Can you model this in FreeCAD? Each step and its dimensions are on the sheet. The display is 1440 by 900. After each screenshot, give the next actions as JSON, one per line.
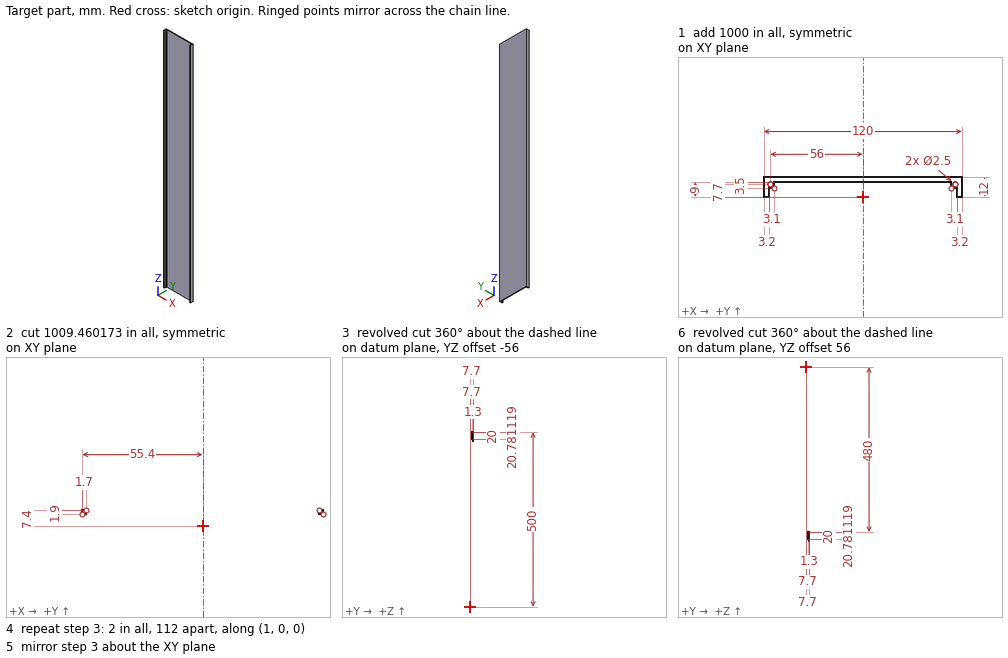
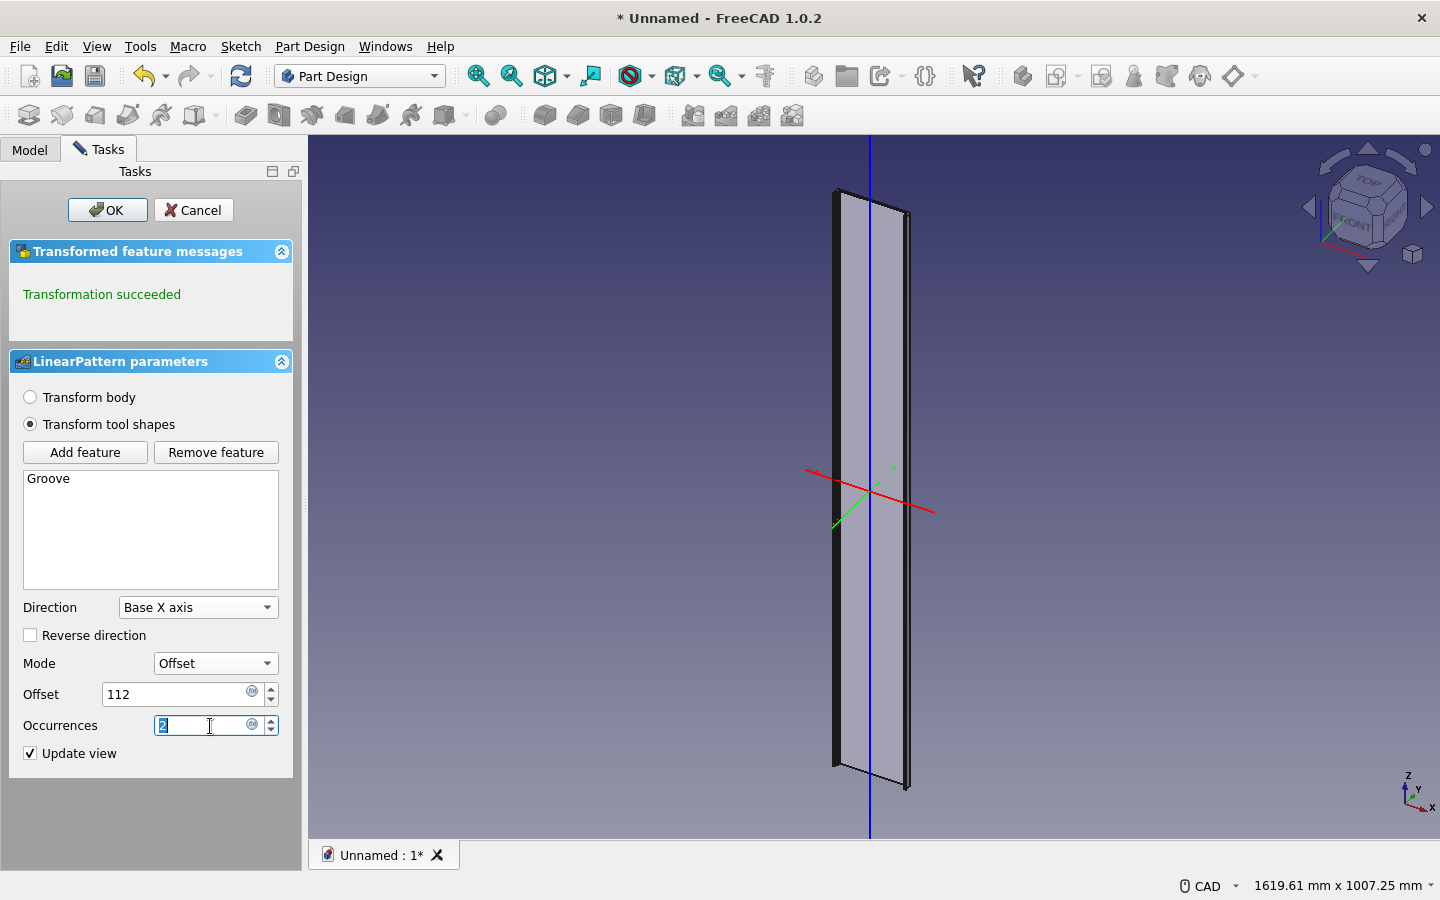
{"action": "type", "text": "2"}
{"action": "key", "text": "Tab"}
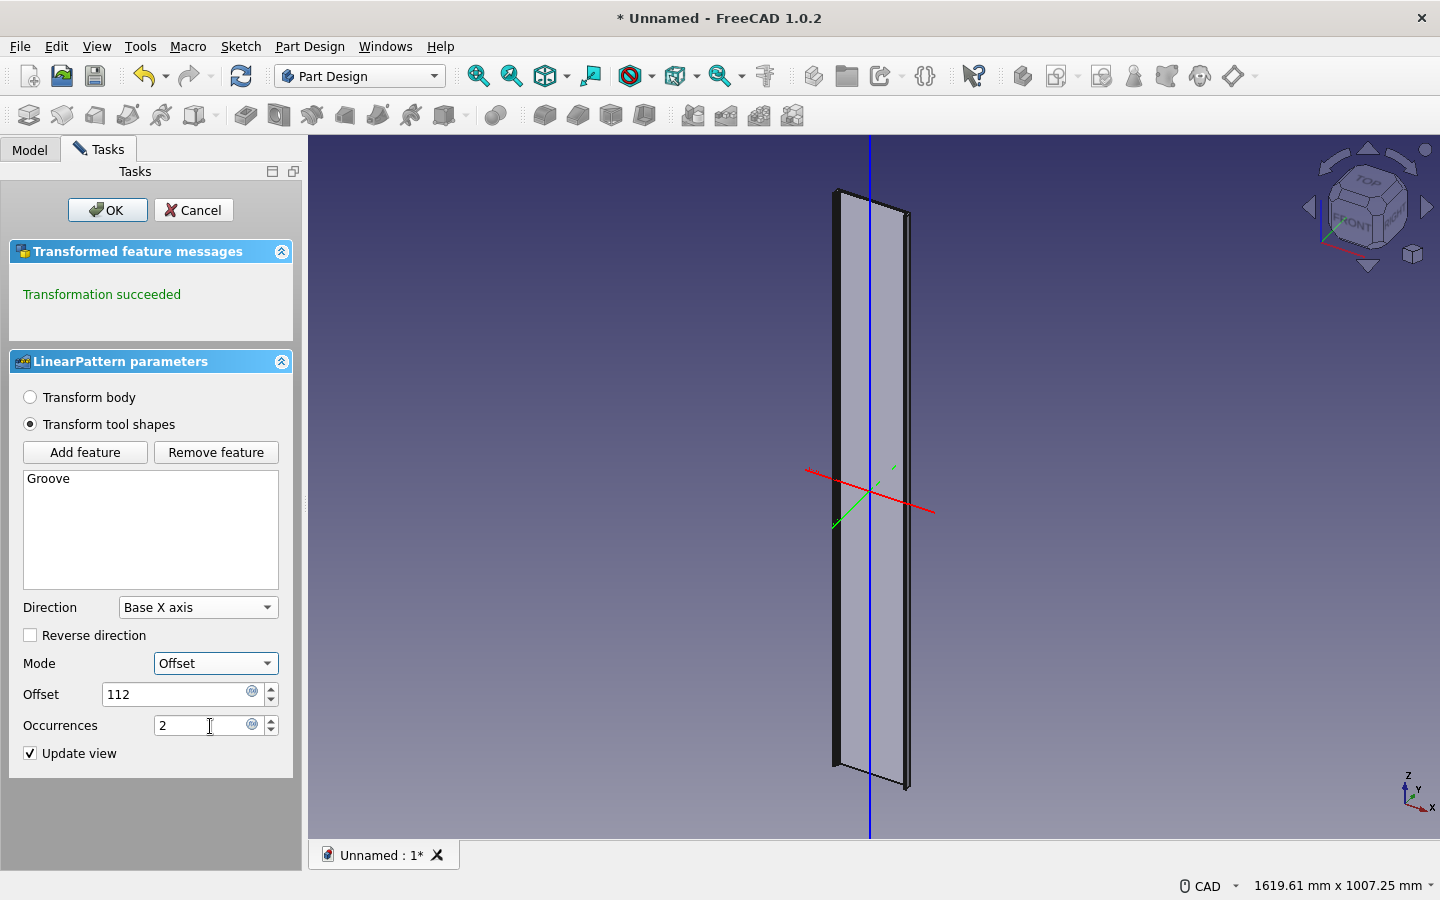
{"action": "left_click", "coordinate": [108, 210]}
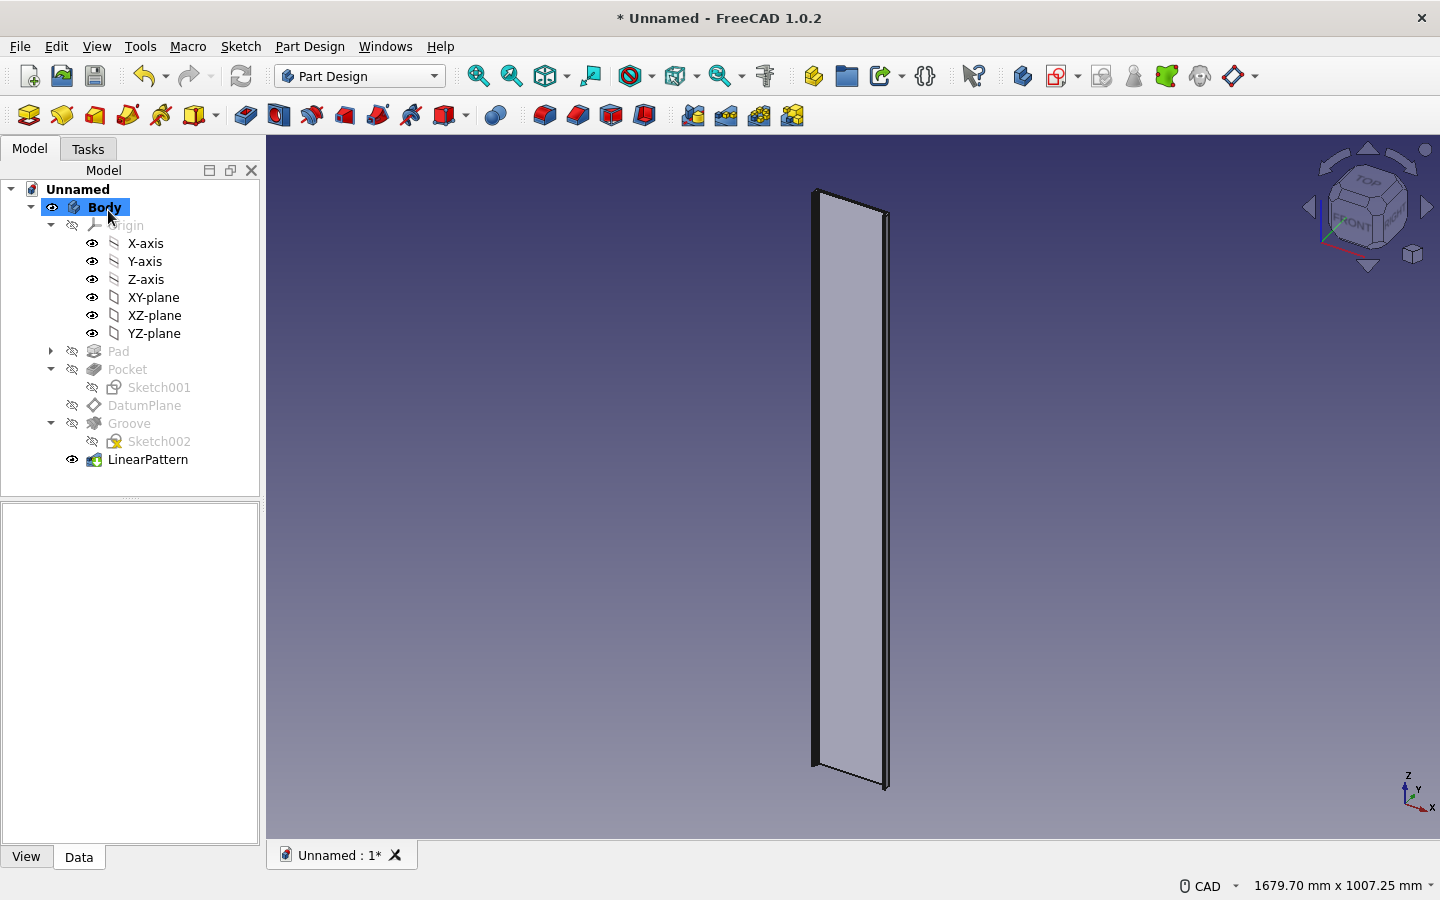
{"action": "left_click", "coordinate": [117, 423]}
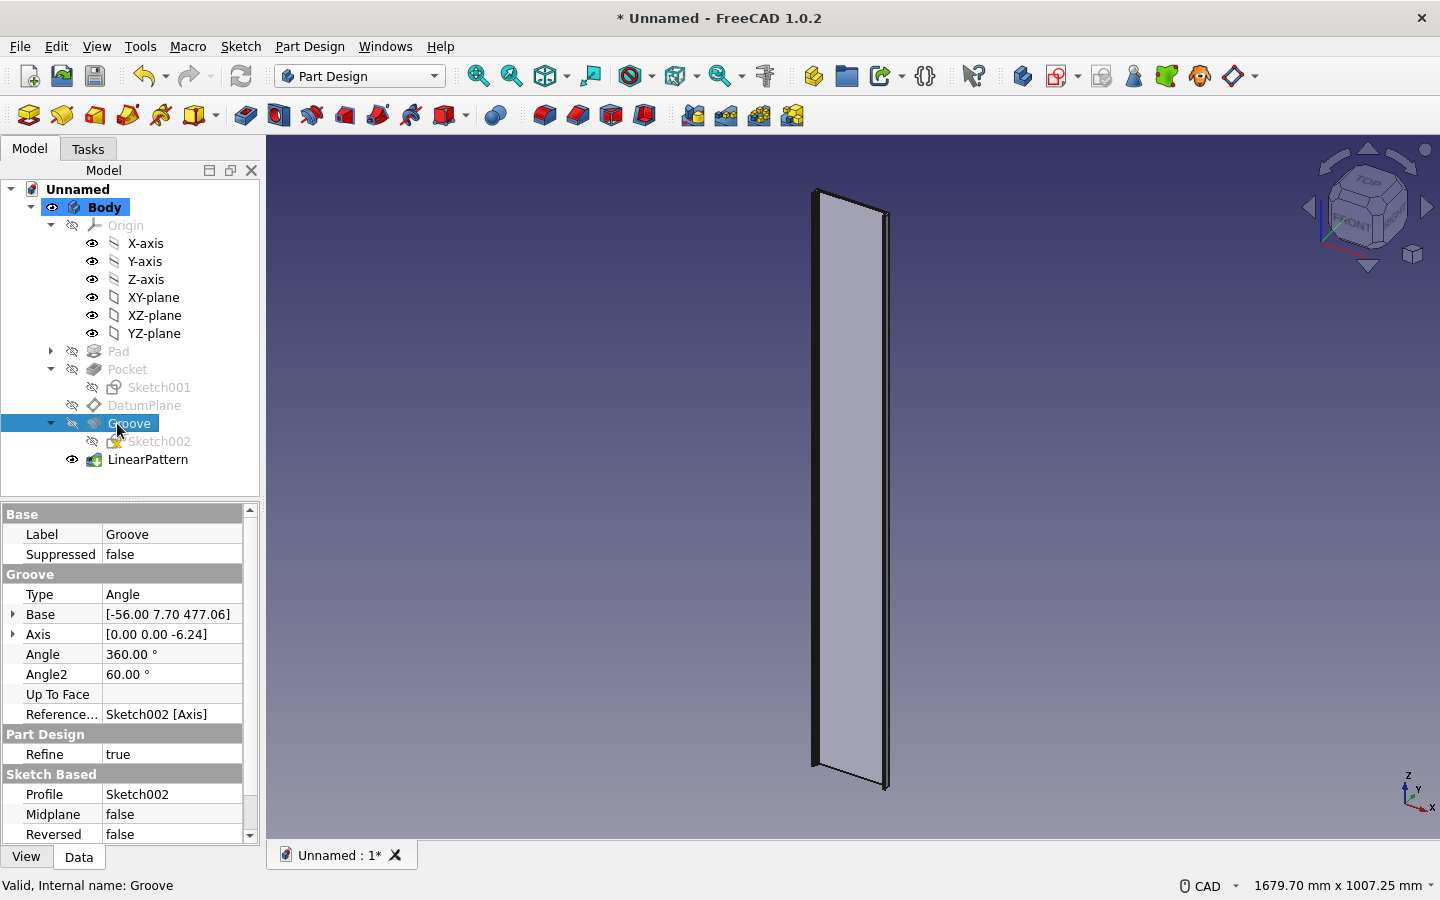
{"action": "left_click", "coordinate": [693, 116]}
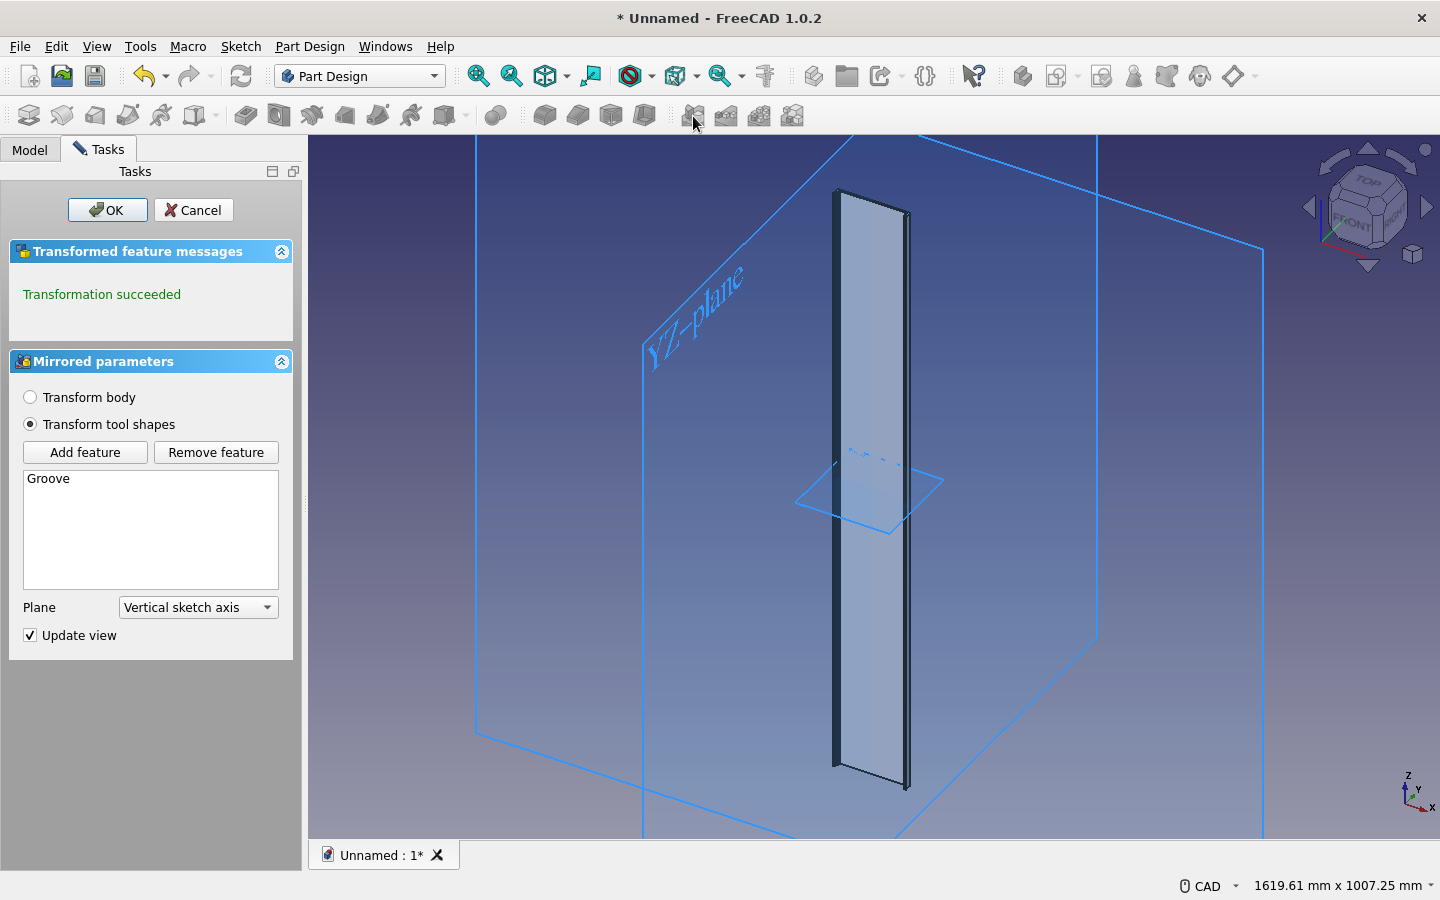
{"action": "left_click", "coordinate": [199, 608]}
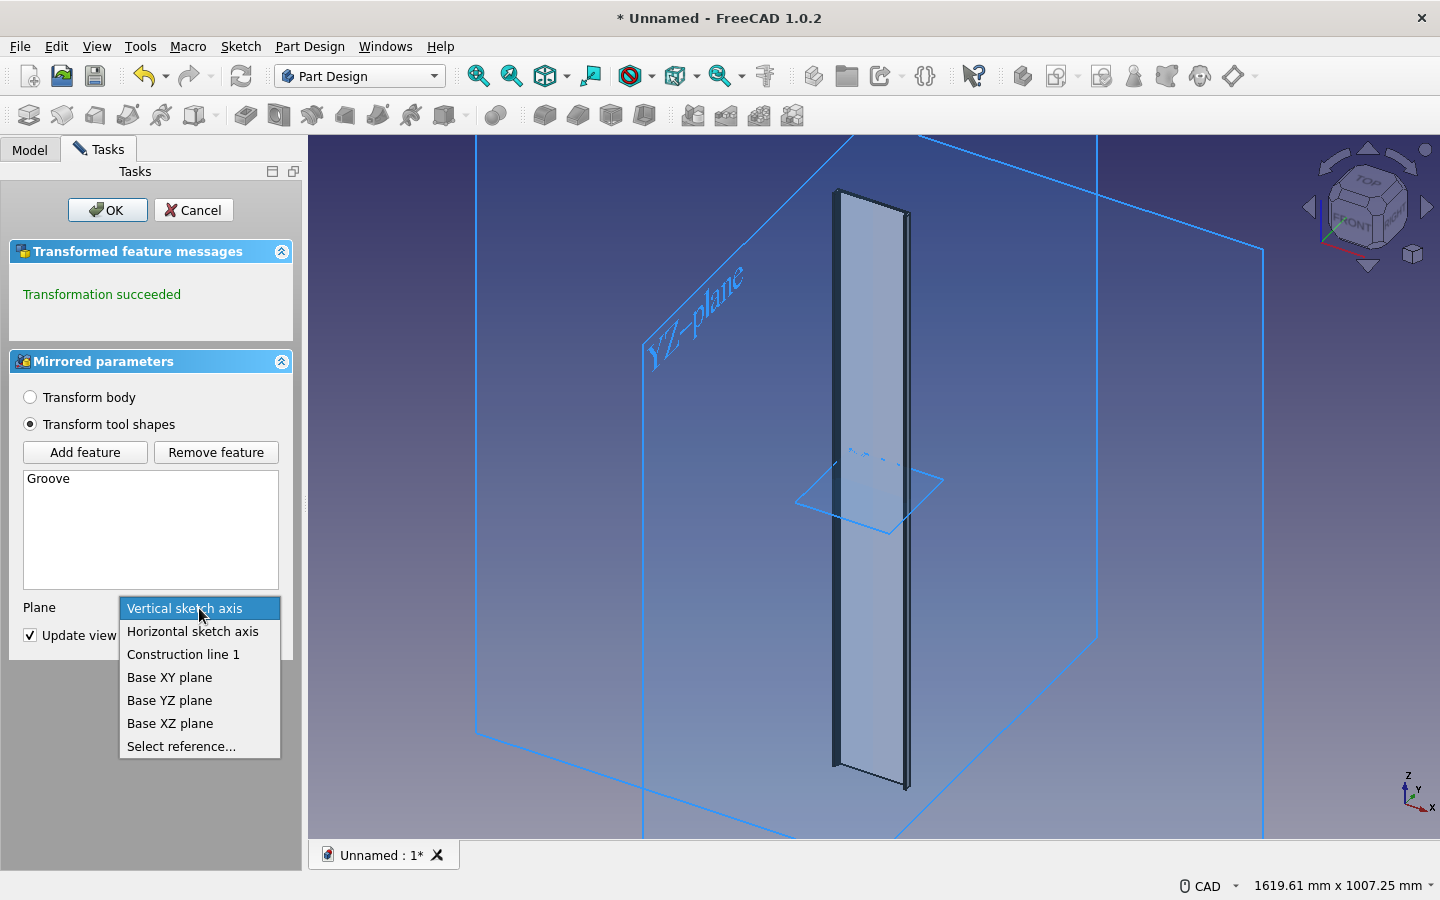
{"action": "left_click", "coordinate": [198, 678]}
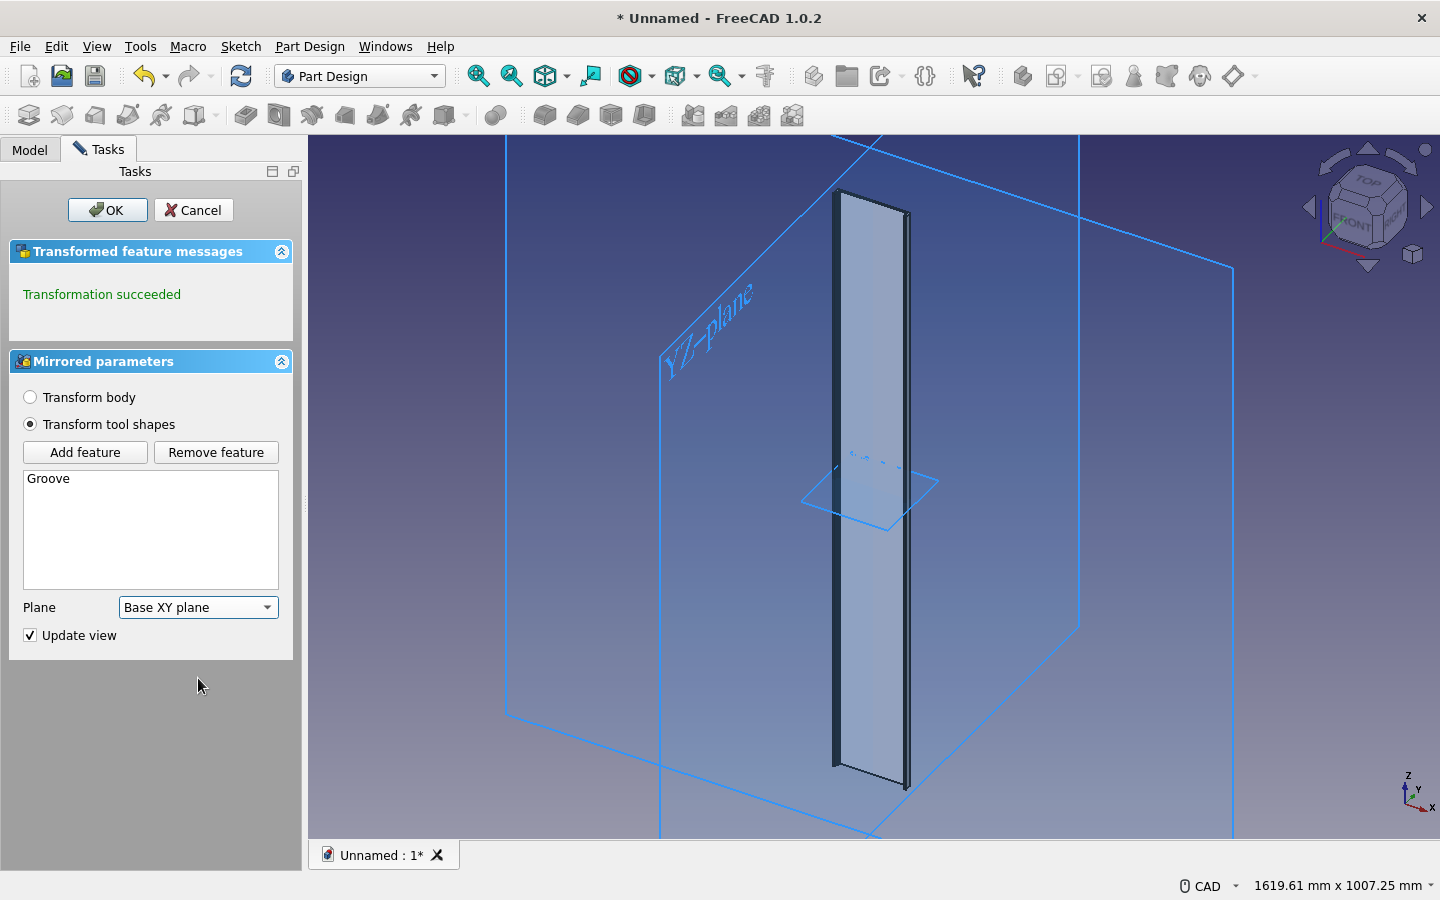
{"action": "left_click", "coordinate": [108, 210]}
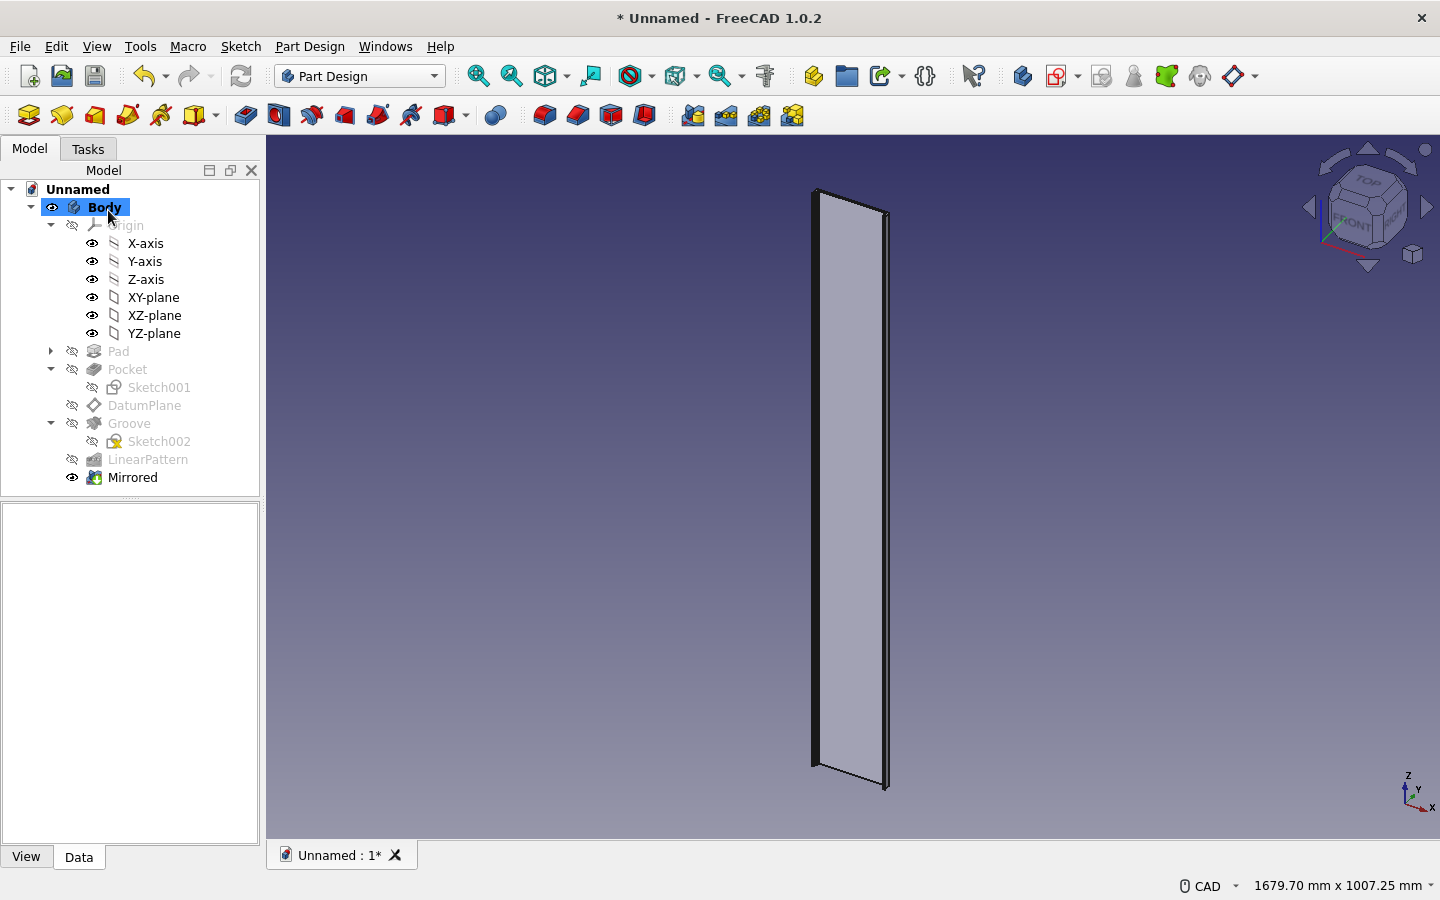
{"action": "left_click", "coordinate": [137, 333]}